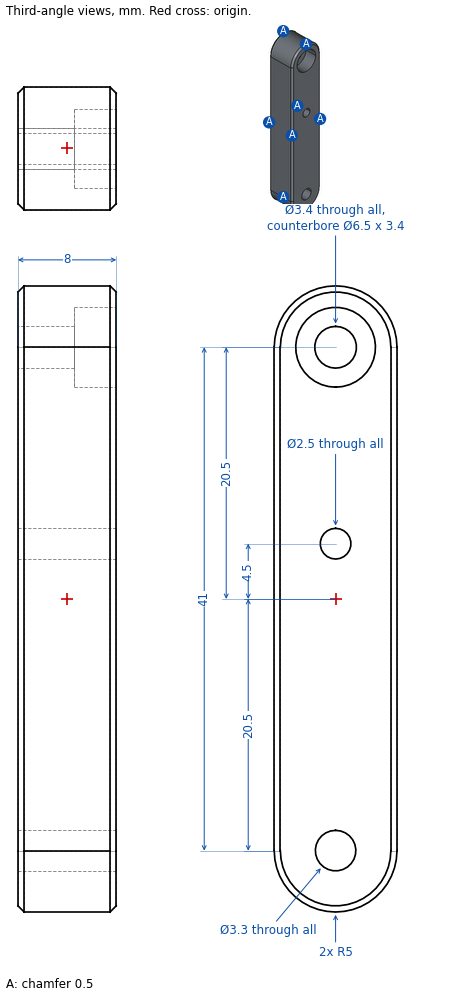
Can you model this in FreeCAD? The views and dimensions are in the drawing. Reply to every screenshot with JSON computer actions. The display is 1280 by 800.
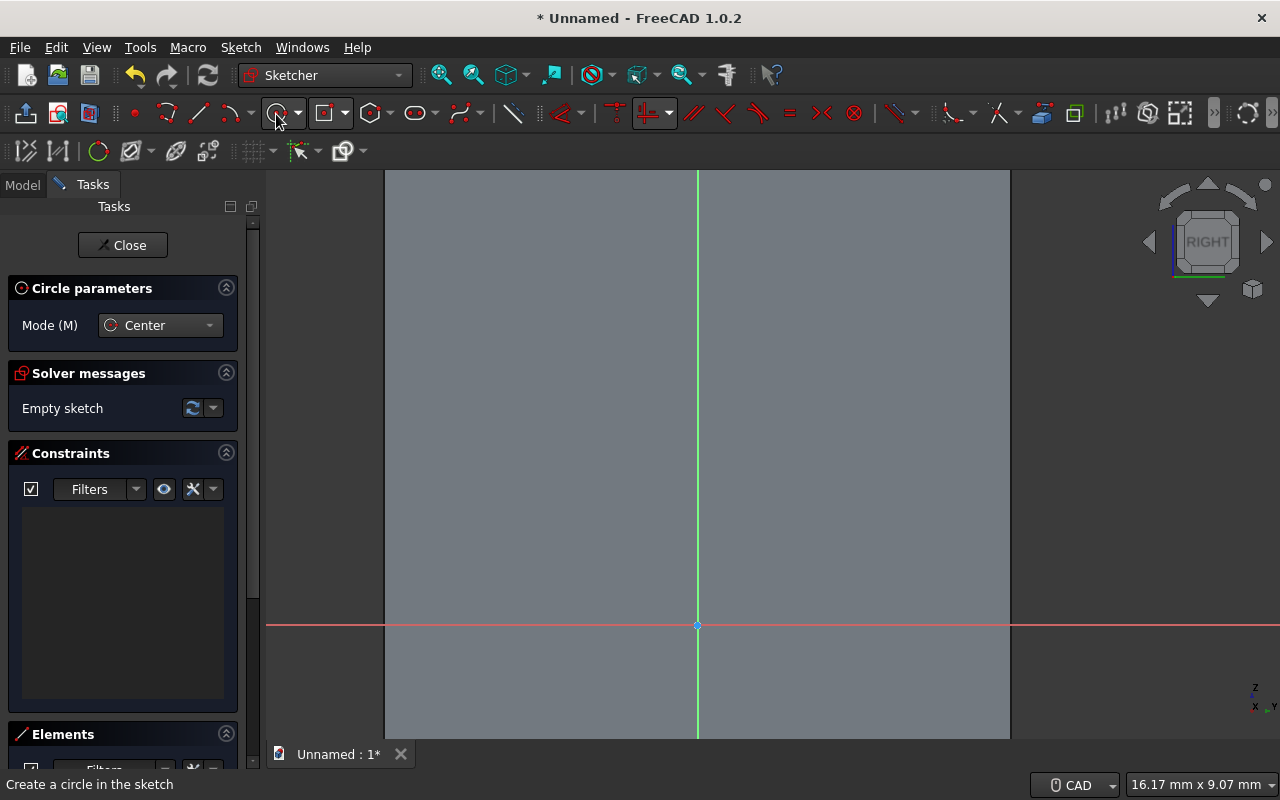
{"action": "left_click", "coordinate": [698, 343]}
{"action": "left_click", "coordinate": [753, 288]}
{"action": "key", "text": "Escape"}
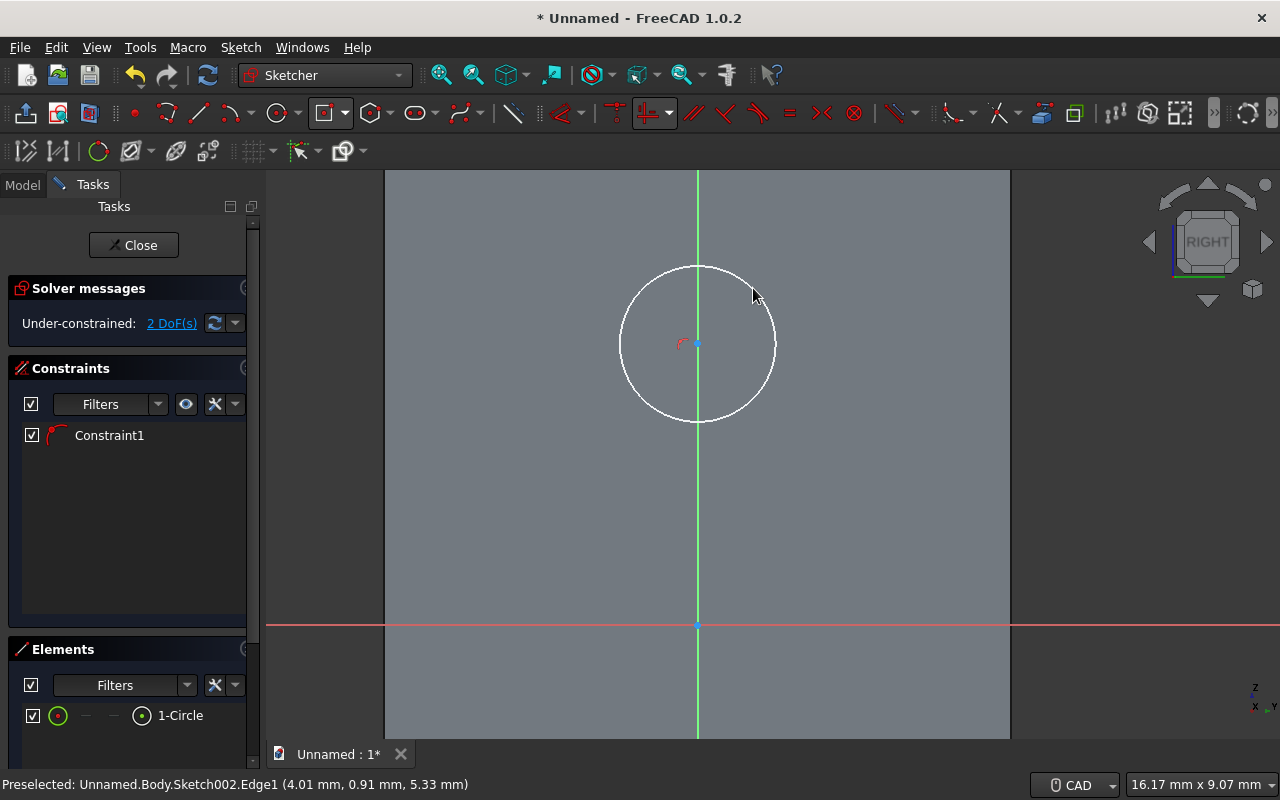
{"action": "key", "text": "d"}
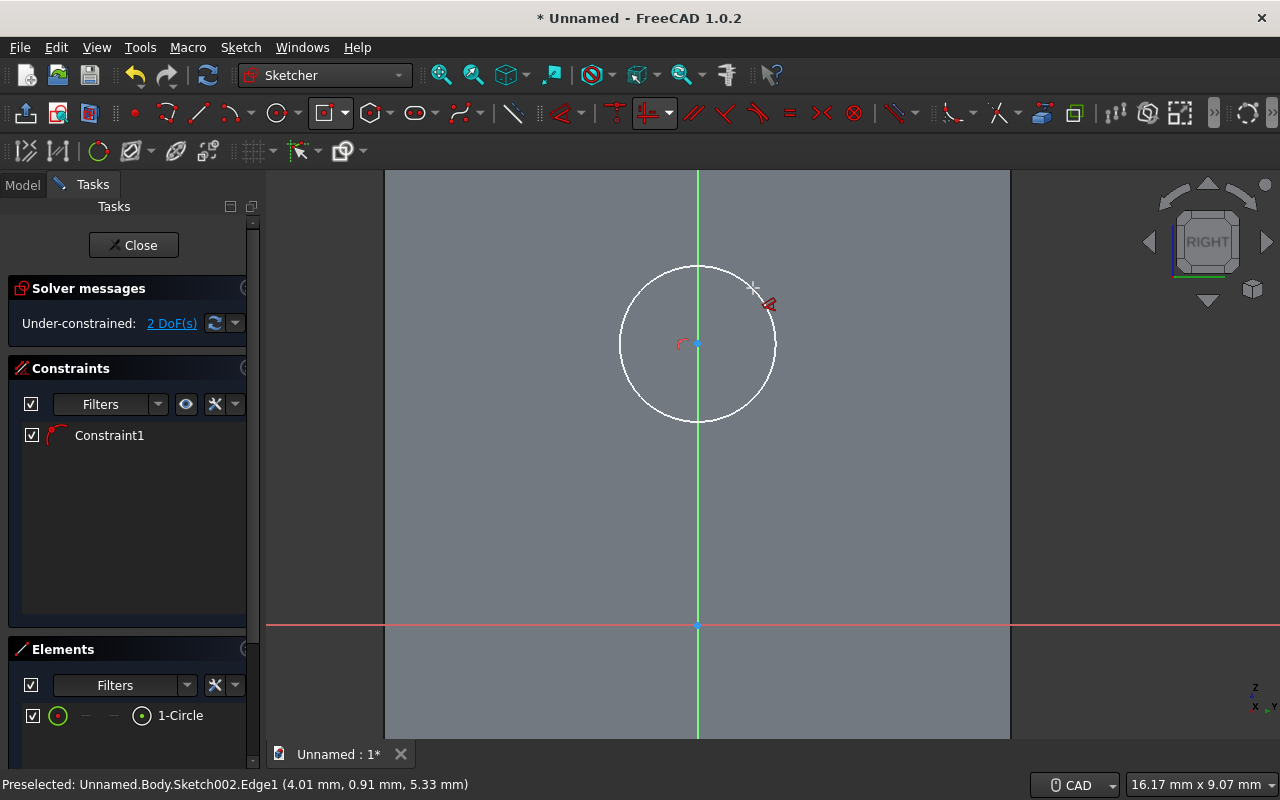
{"action": "left_click", "coordinate": [753, 289]}
{"action": "left_click", "coordinate": [776, 266]}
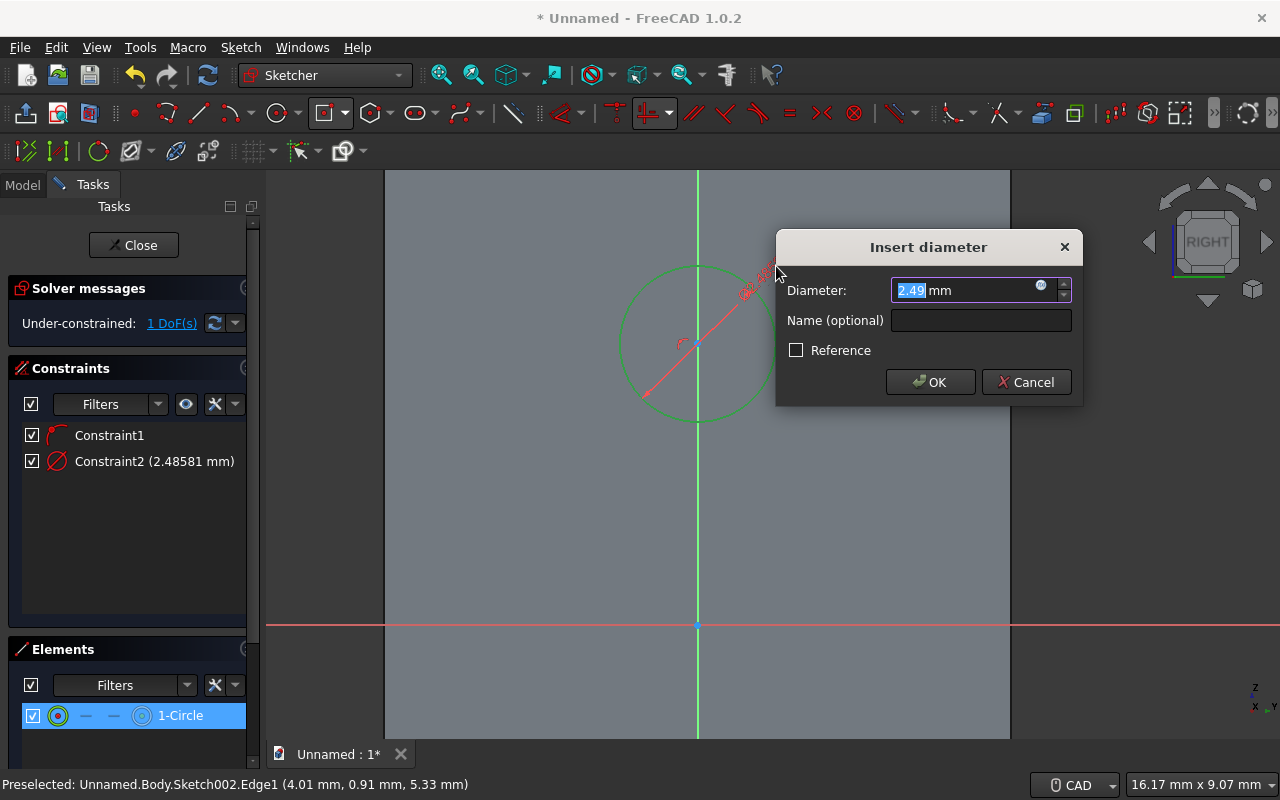
{"action": "type", "text": "2.5"}
{"action": "key", "text": "Return"}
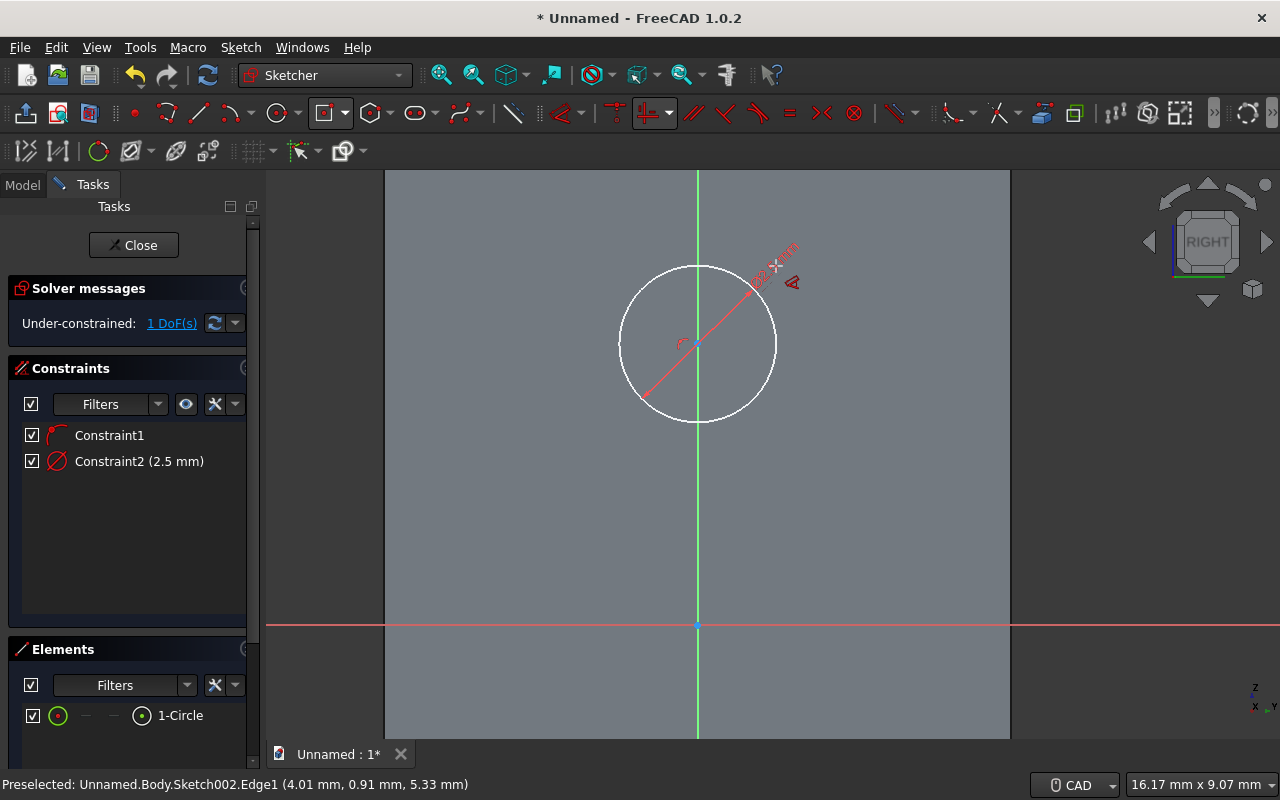
{"action": "left_click", "coordinate": [698, 344]}
{"action": "left_click", "coordinate": [732, 485]}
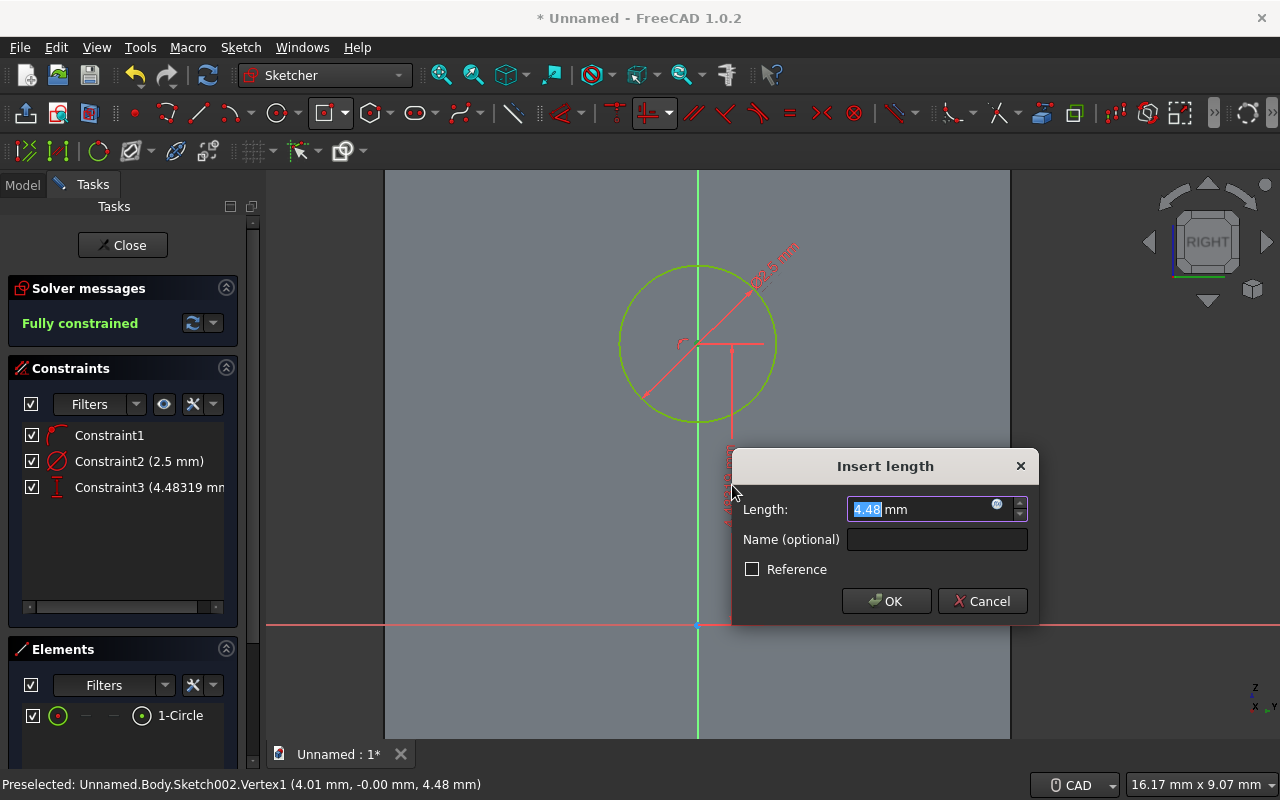
{"action": "type", "text": "4.5"}
{"action": "key", "text": "Return"}
{"action": "key", "text": "Escape"}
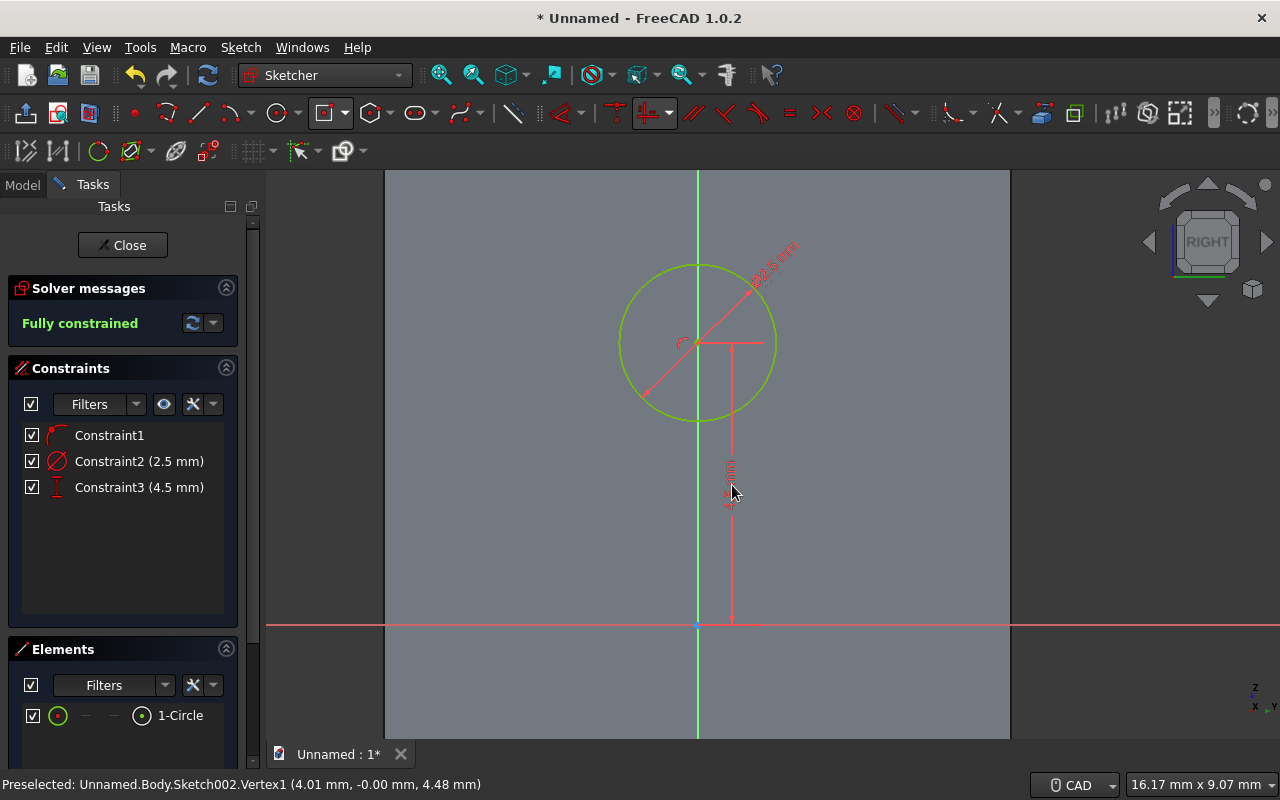
{"action": "left_click", "coordinate": [123, 245]}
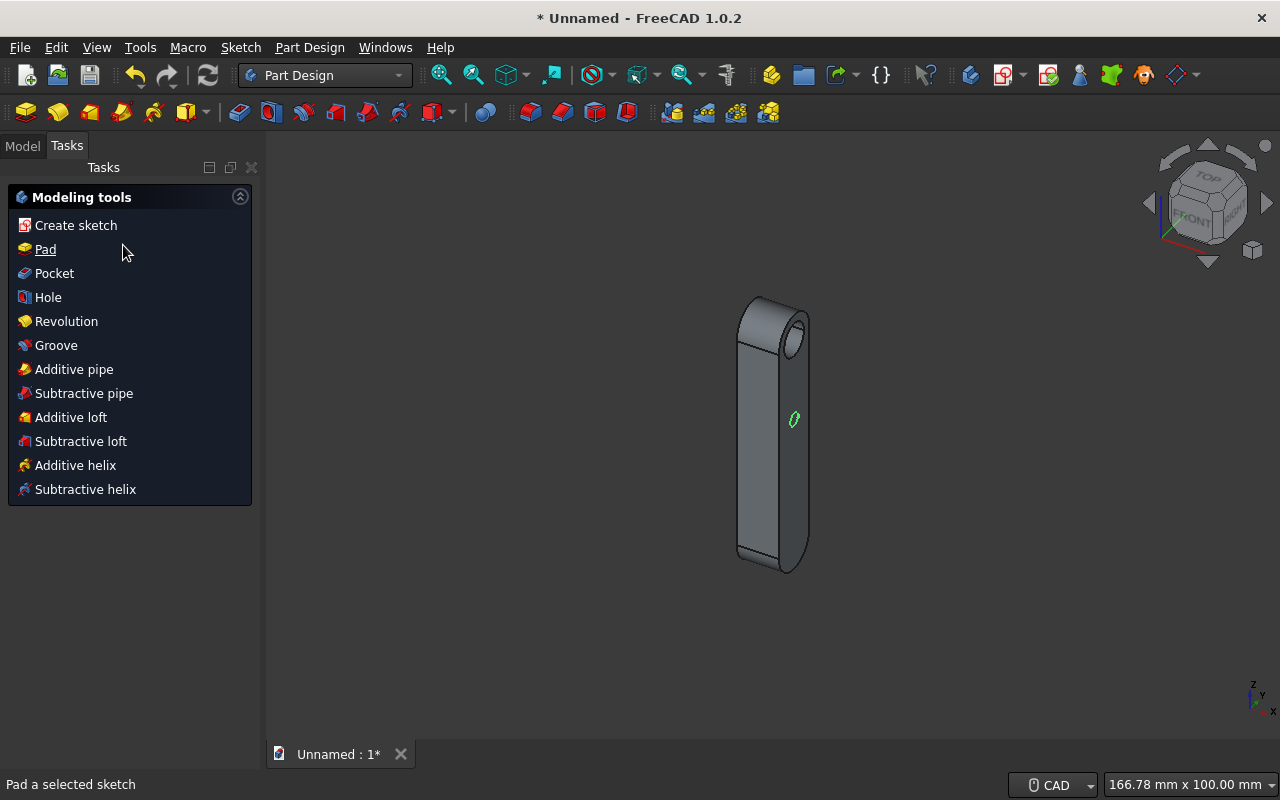
{"action": "left_click", "coordinate": [272, 112]}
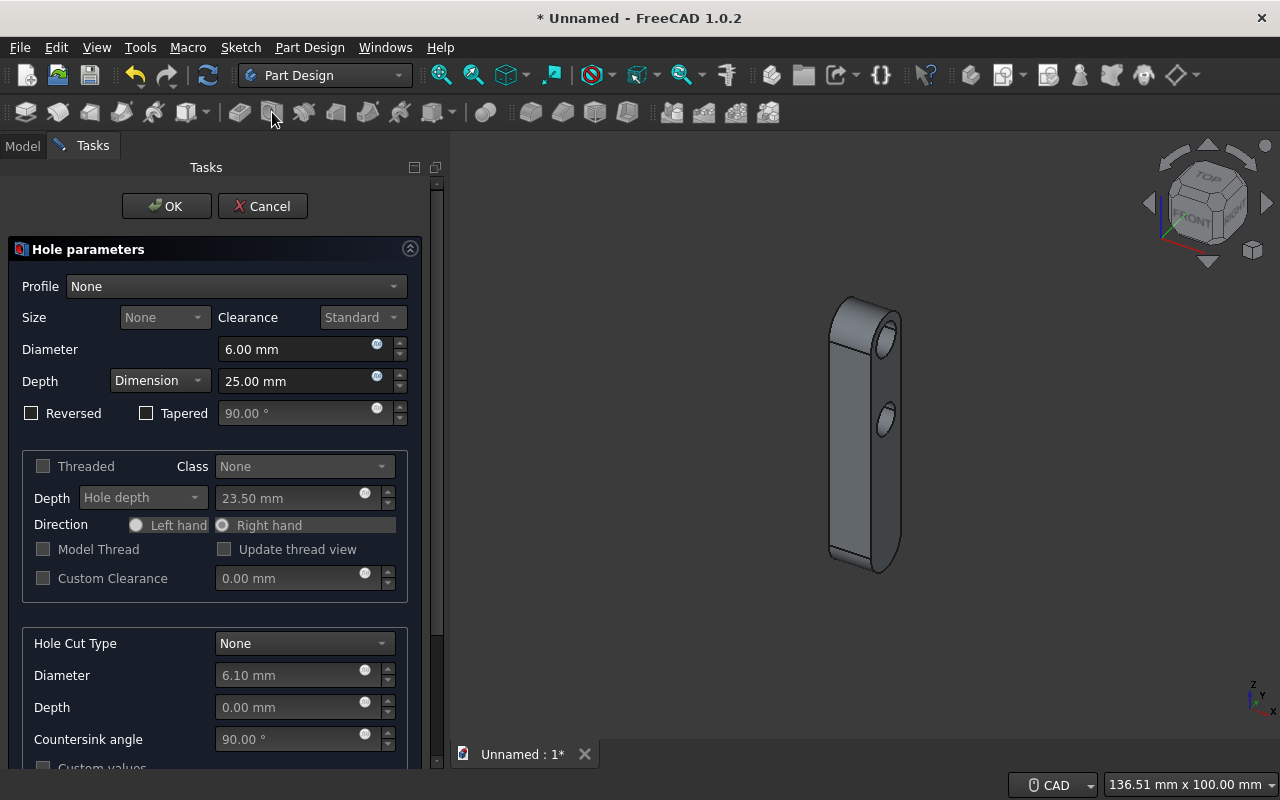
{"action": "triple_click", "coordinate": [305, 349]}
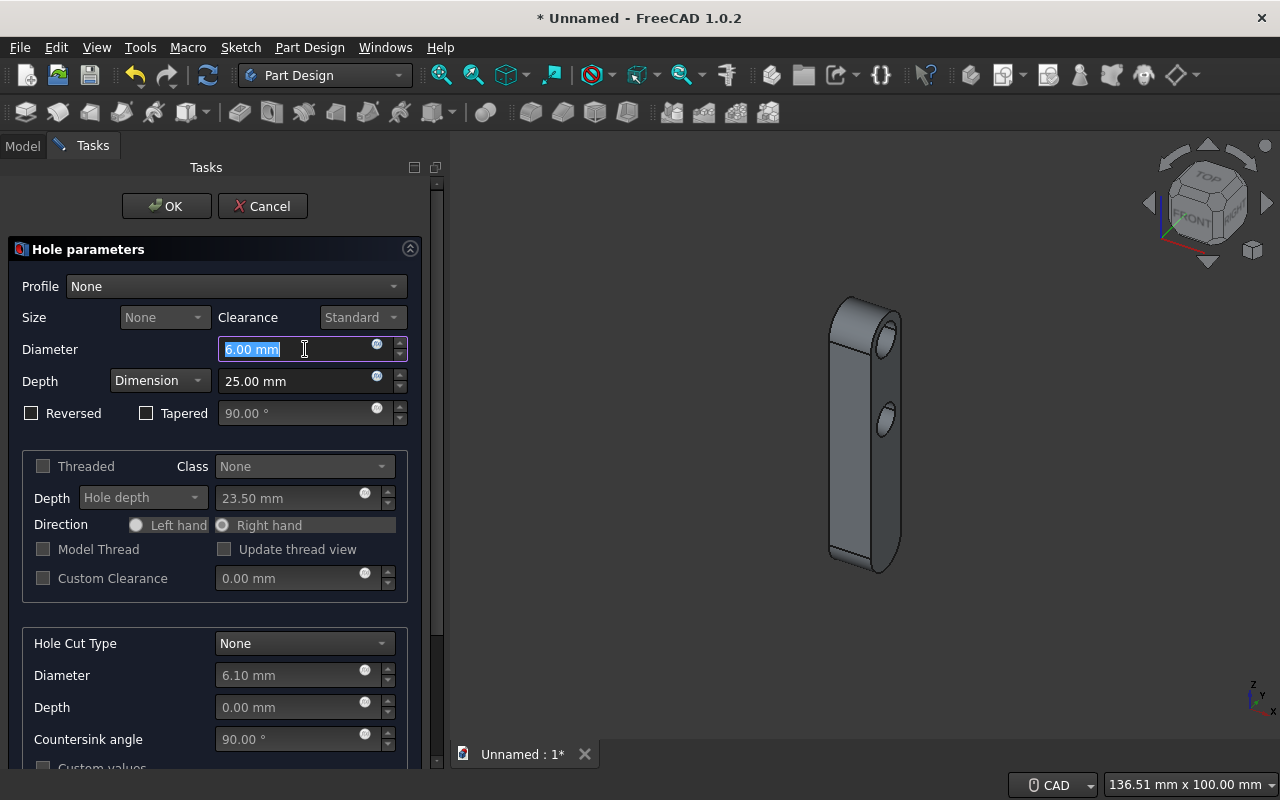
{"action": "type", "text": "2.5"}
{"action": "key", "text": "Tab"}